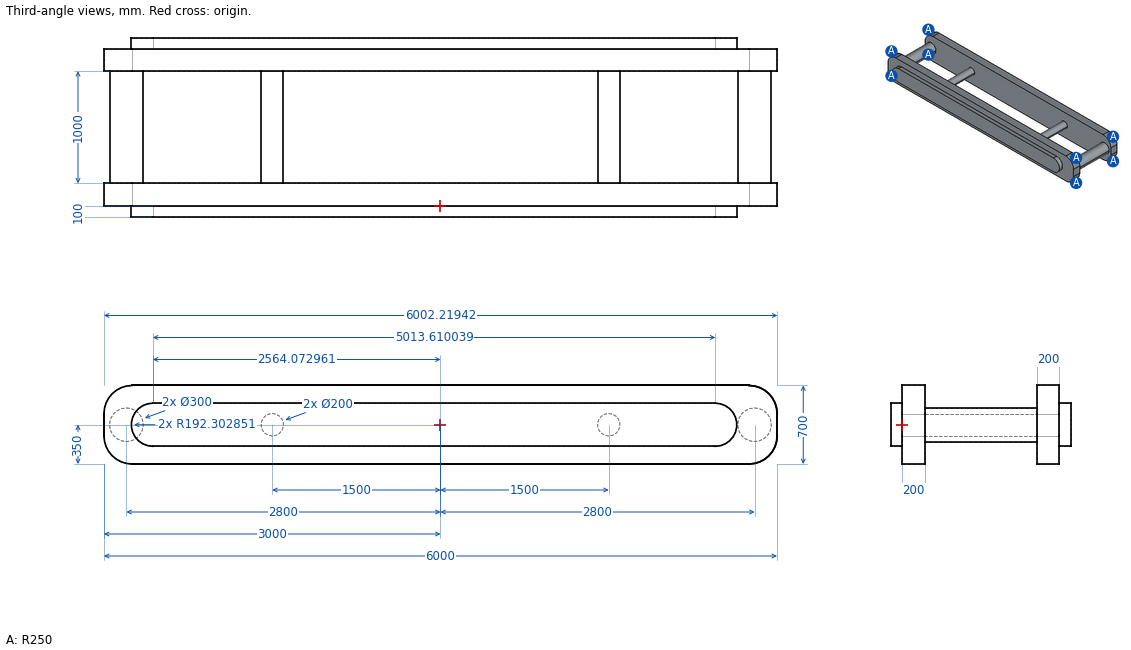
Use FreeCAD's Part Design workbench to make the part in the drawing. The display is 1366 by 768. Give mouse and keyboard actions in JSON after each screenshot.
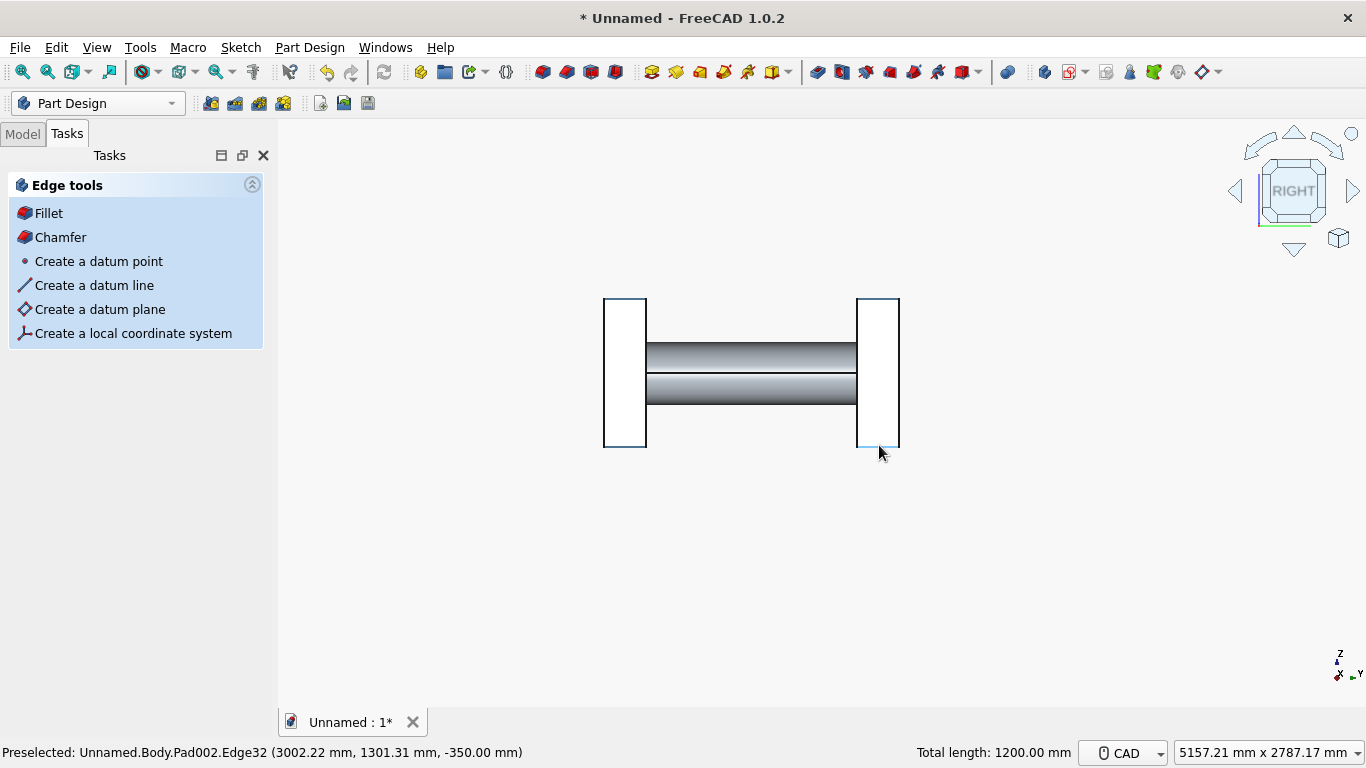
{"action": "key", "text": "v f"}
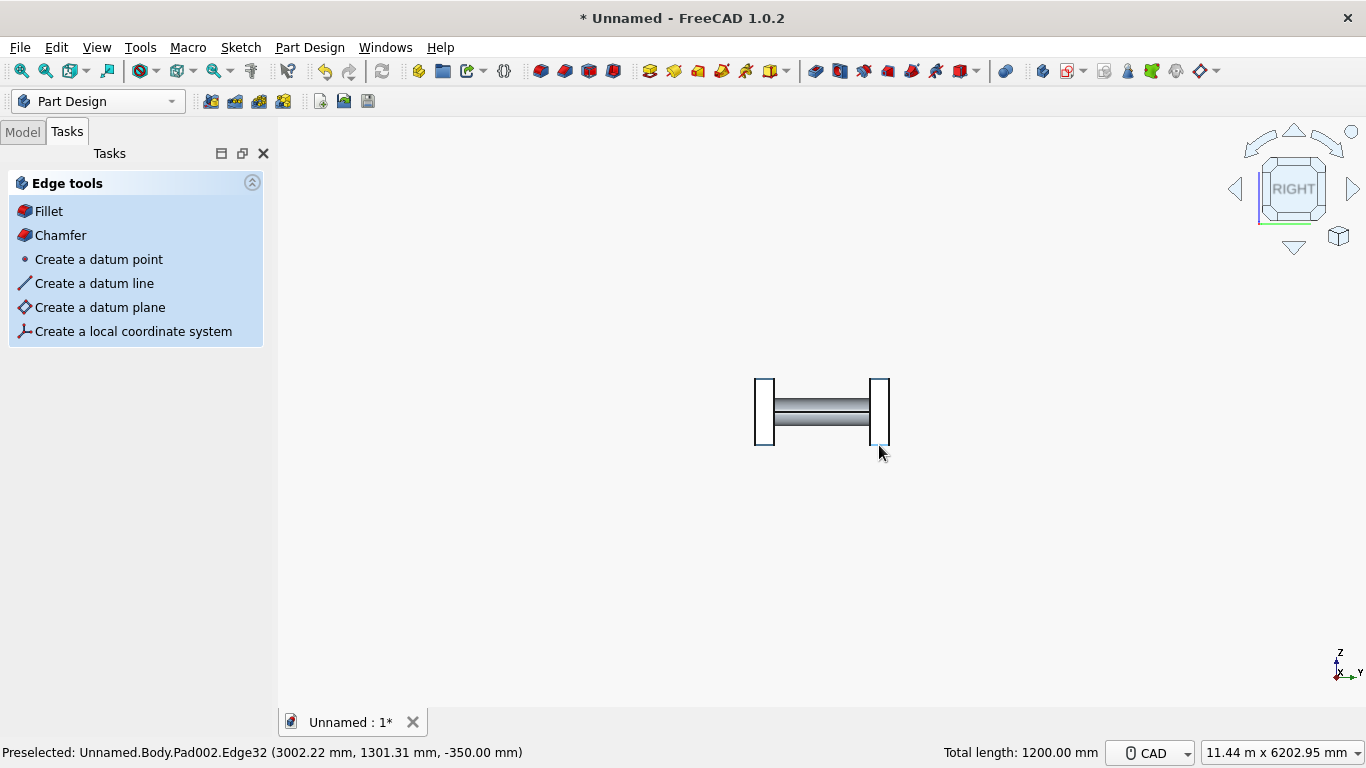
{"action": "key", "text": "5"}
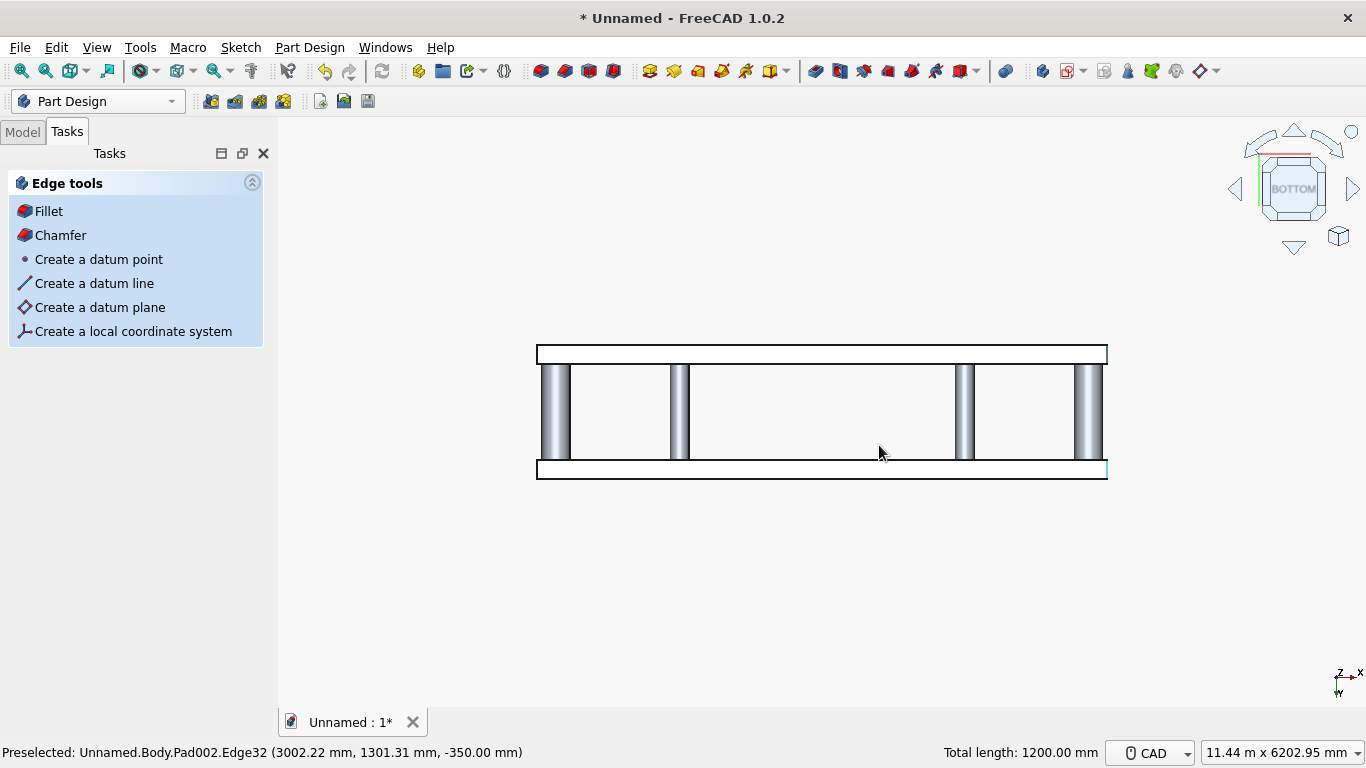
{"action": "left_click", "coordinate": [537, 468], "text": "ctrl"}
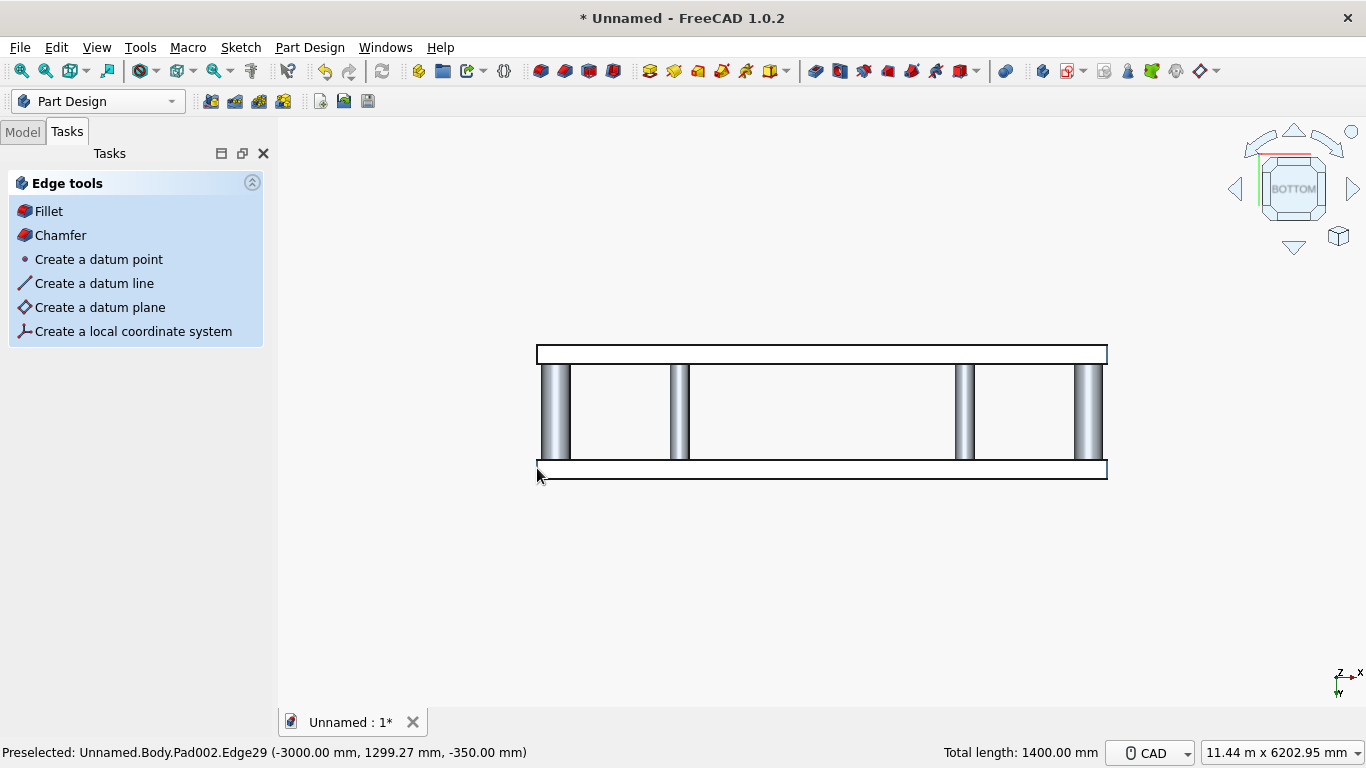
{"action": "left_click", "coordinate": [537, 354], "text": "ctrl"}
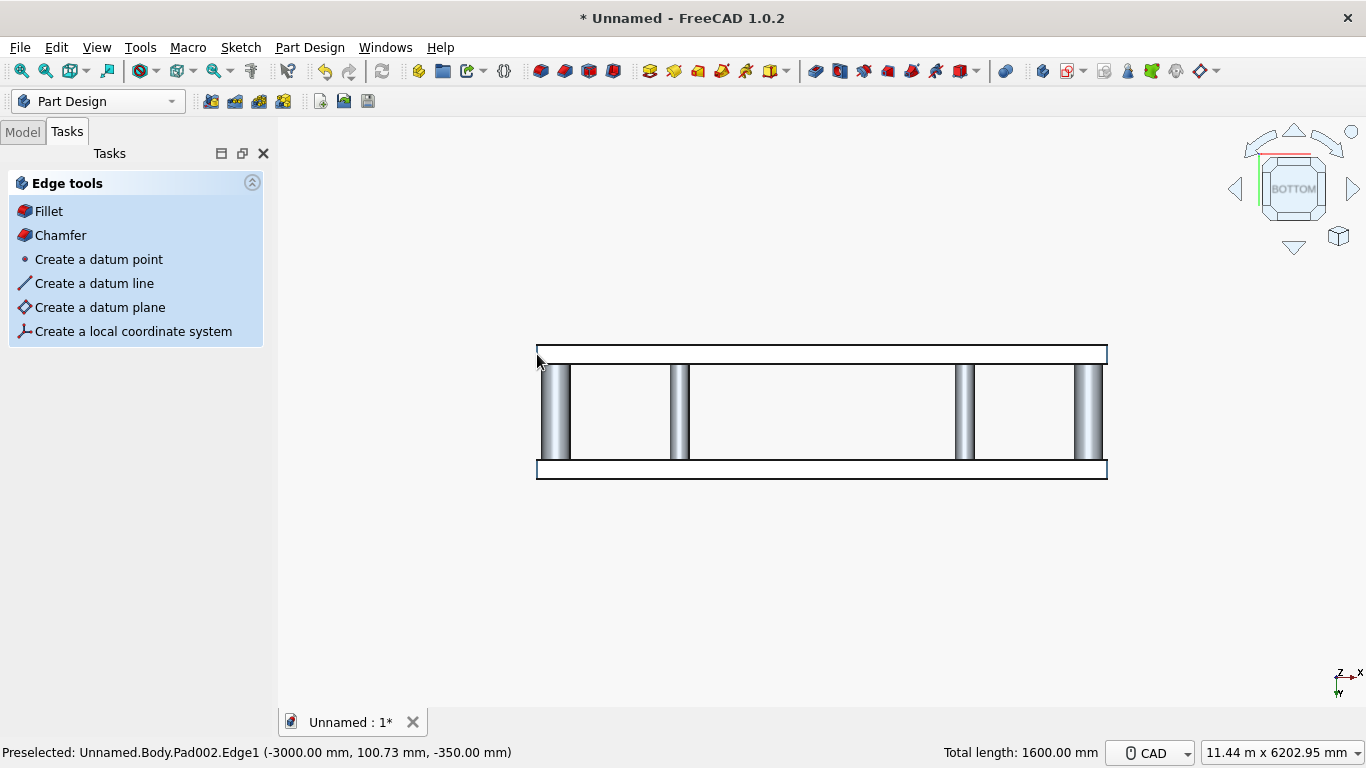
{"action": "left_click", "coordinate": [542, 72]}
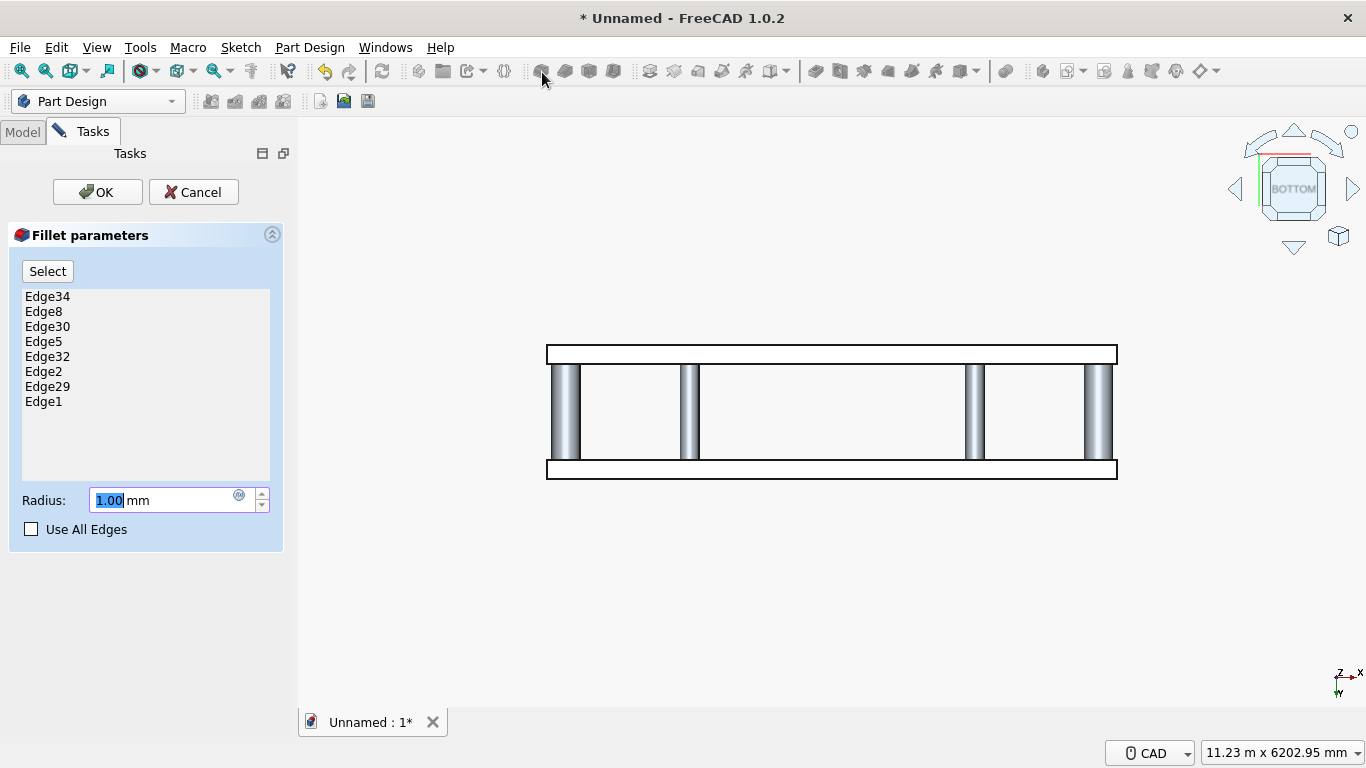
{"action": "type", "text": "250"}
{"action": "key", "text": "Tab"}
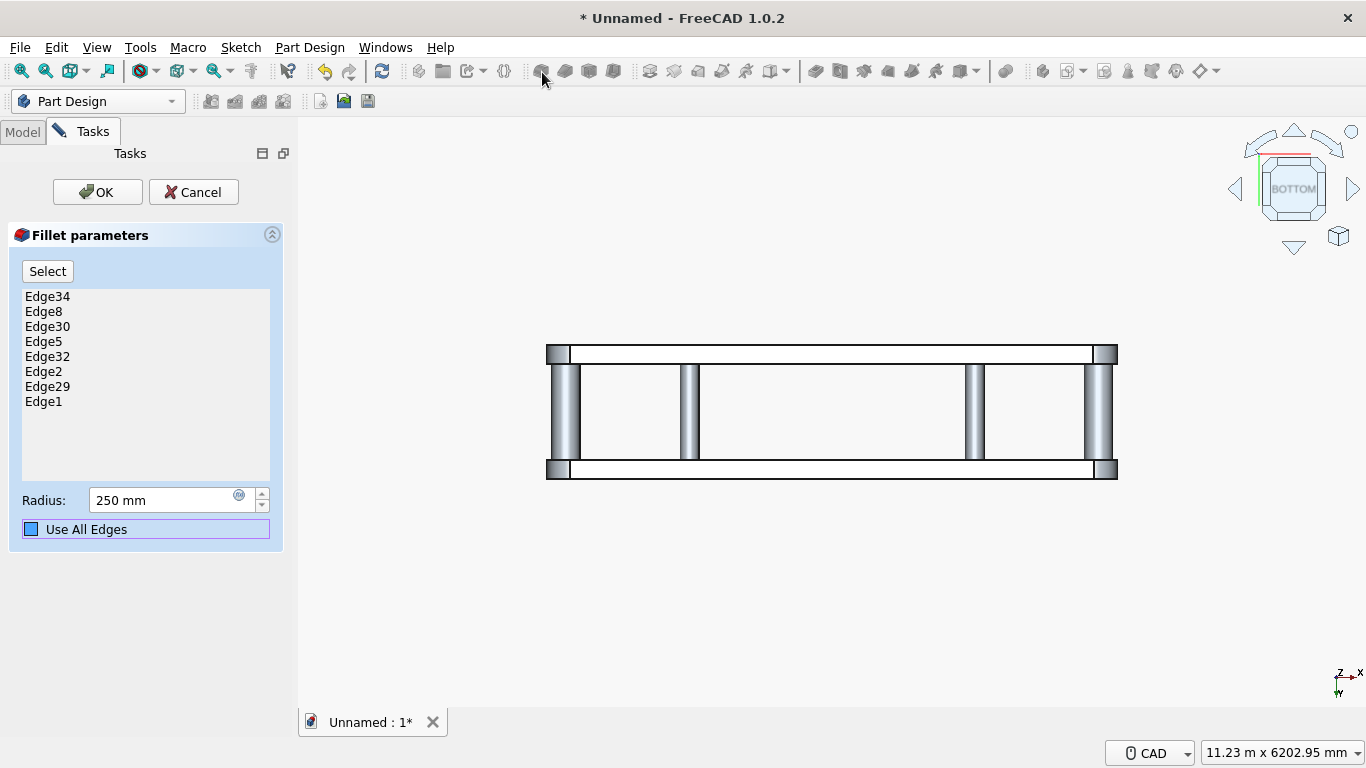
{"action": "left_click", "coordinate": [98, 192]}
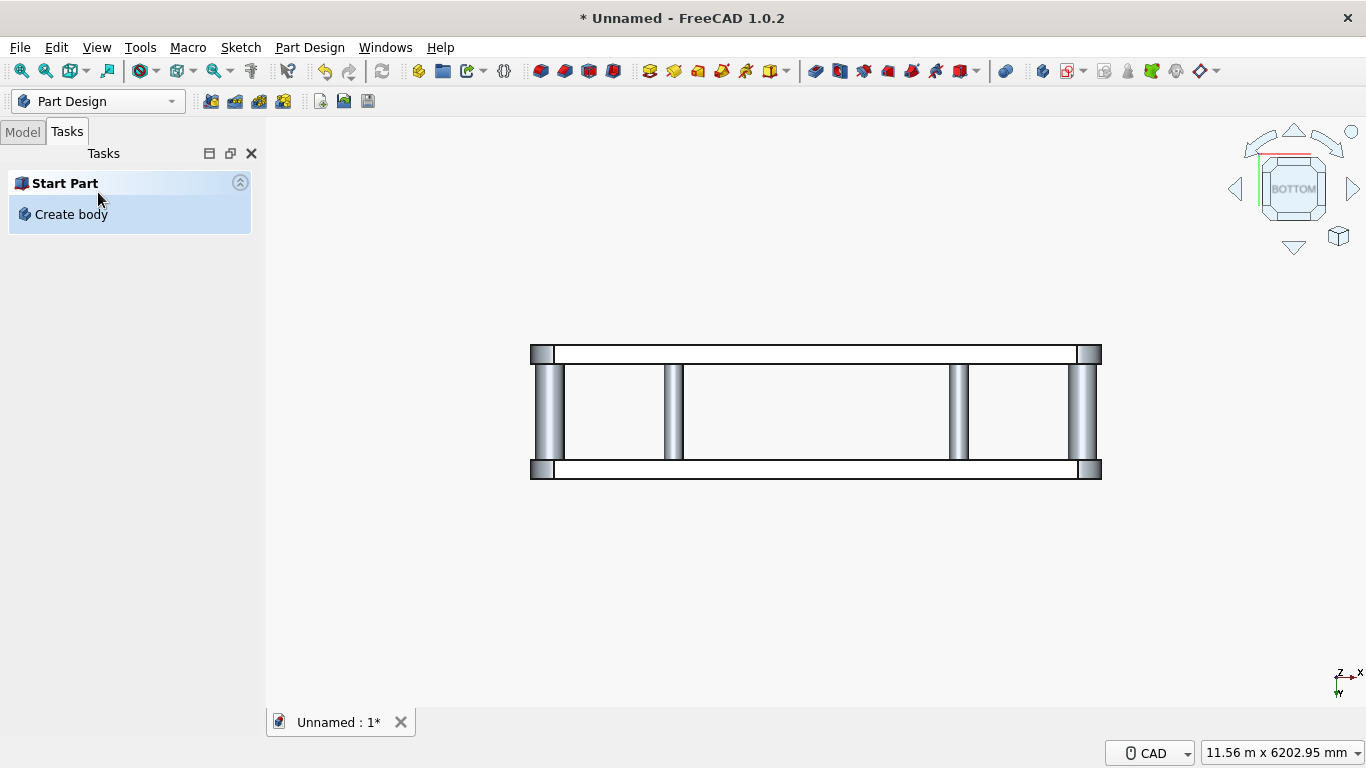
{"action": "key", "text": "0"}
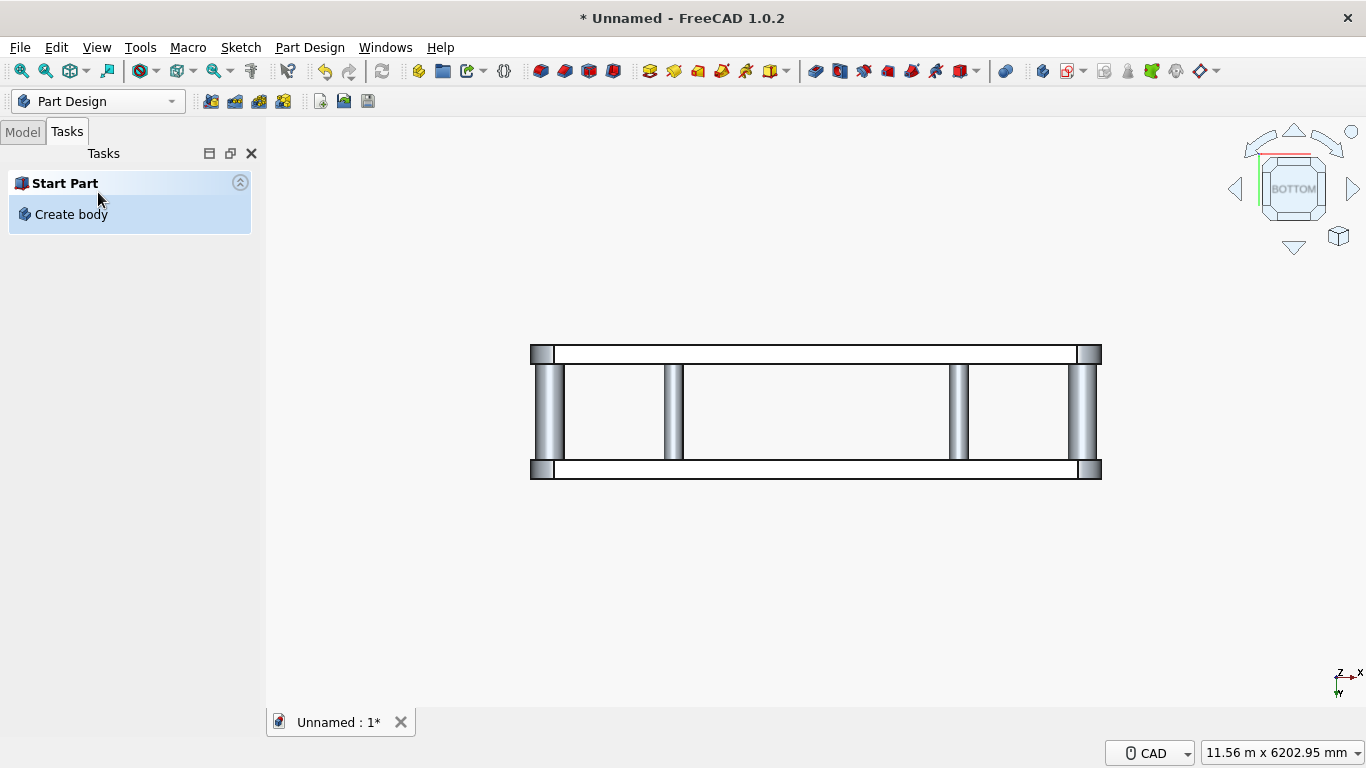
{"action": "left_click", "coordinate": [942, 538]}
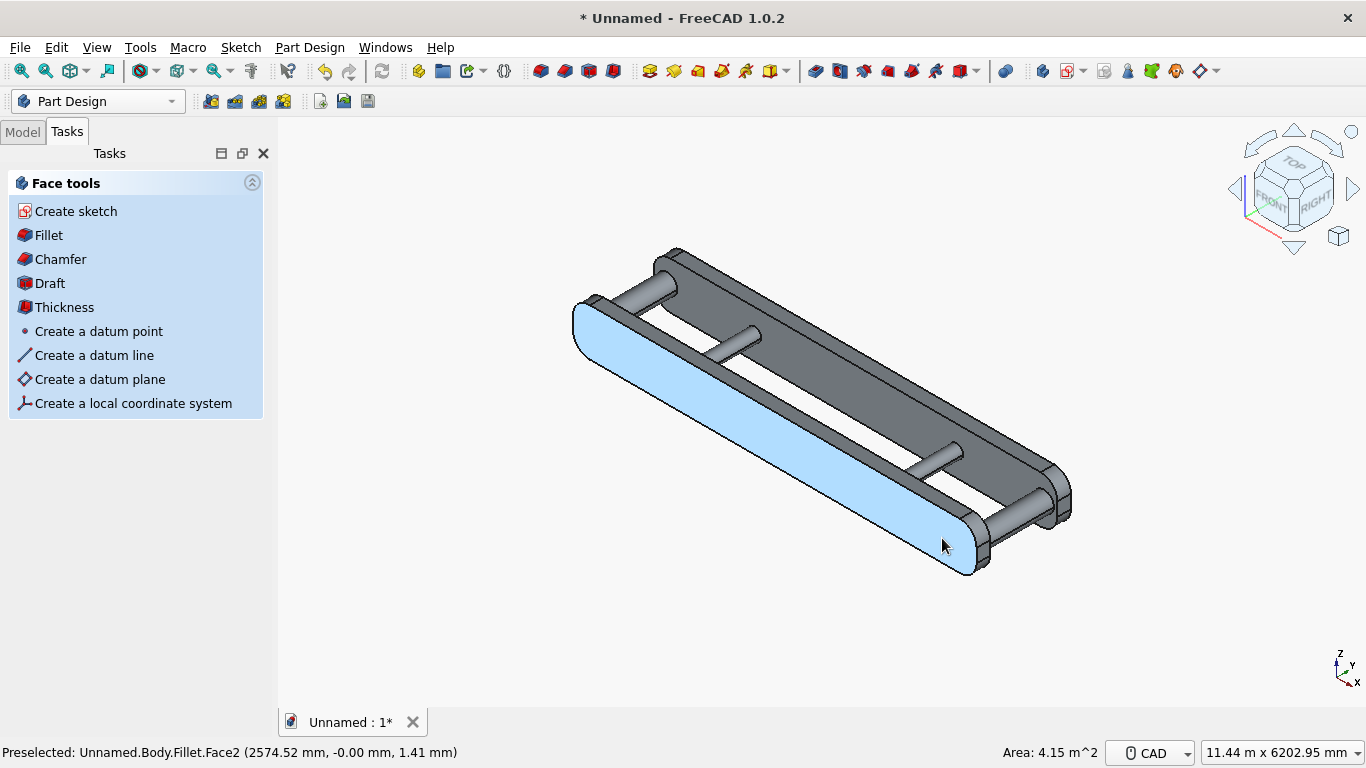
{"action": "left_click", "coordinate": [1068, 72]}